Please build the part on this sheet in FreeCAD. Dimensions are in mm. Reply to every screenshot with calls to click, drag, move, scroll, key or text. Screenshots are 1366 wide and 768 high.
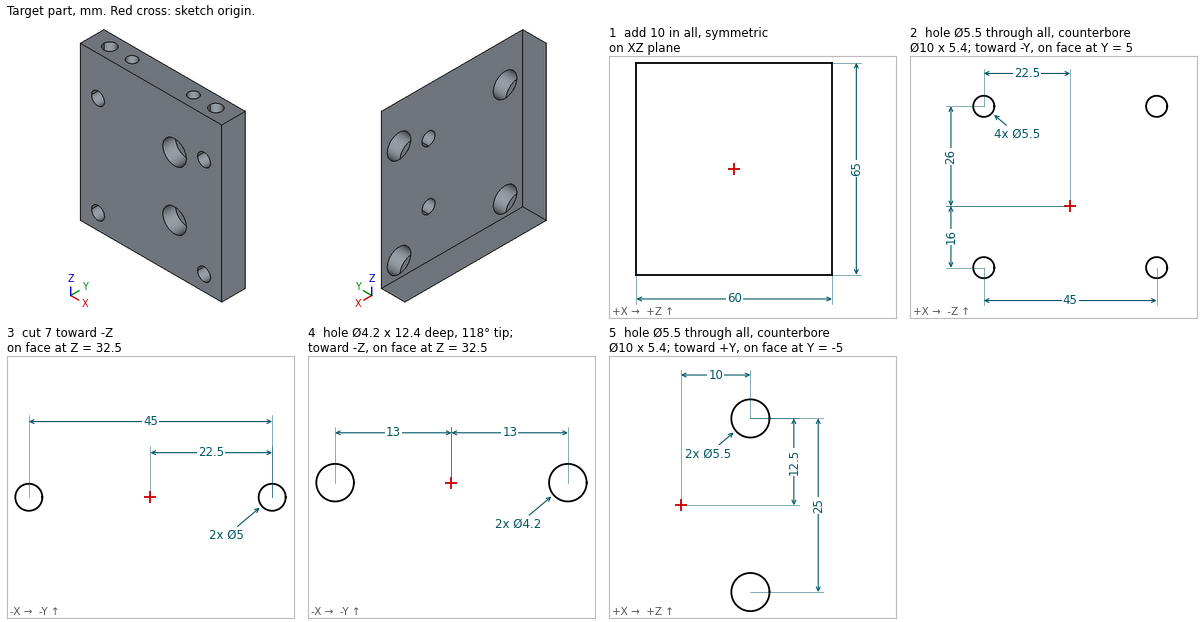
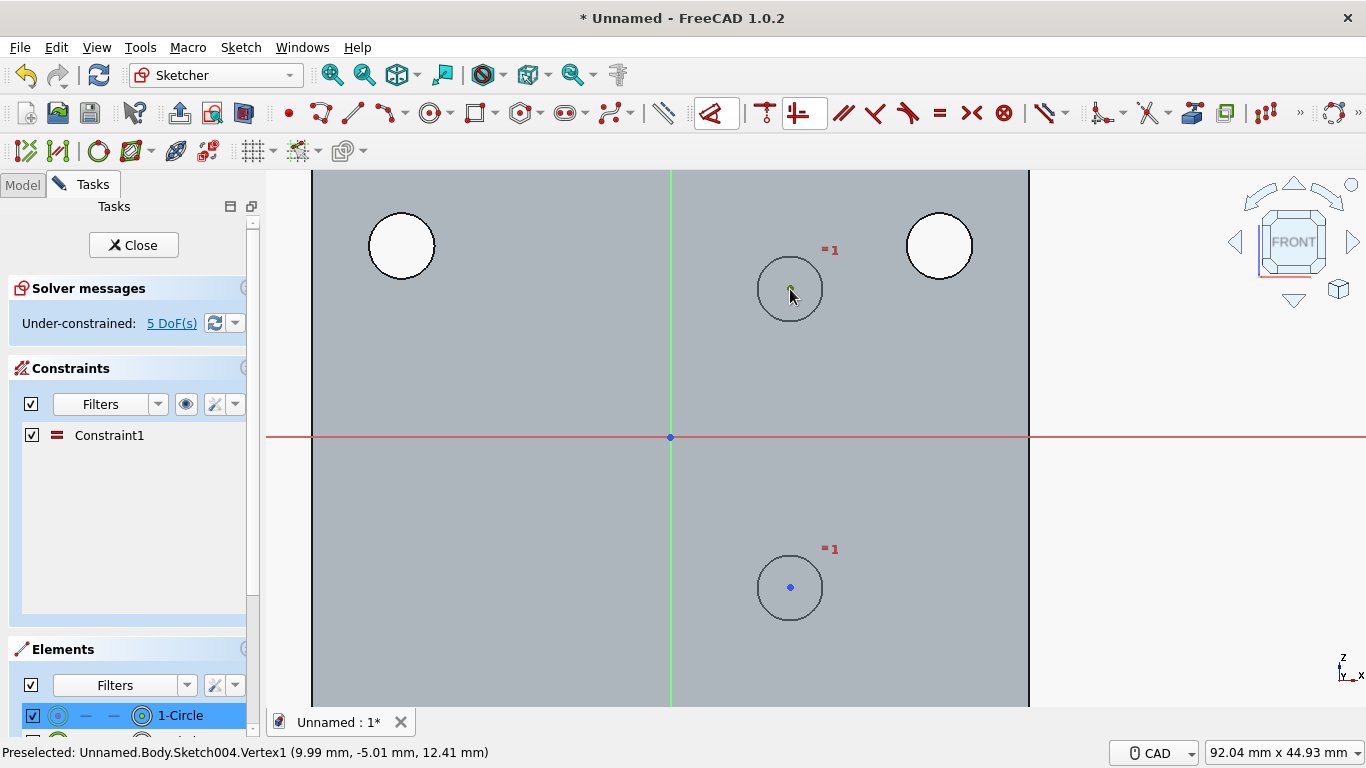
click(790, 588)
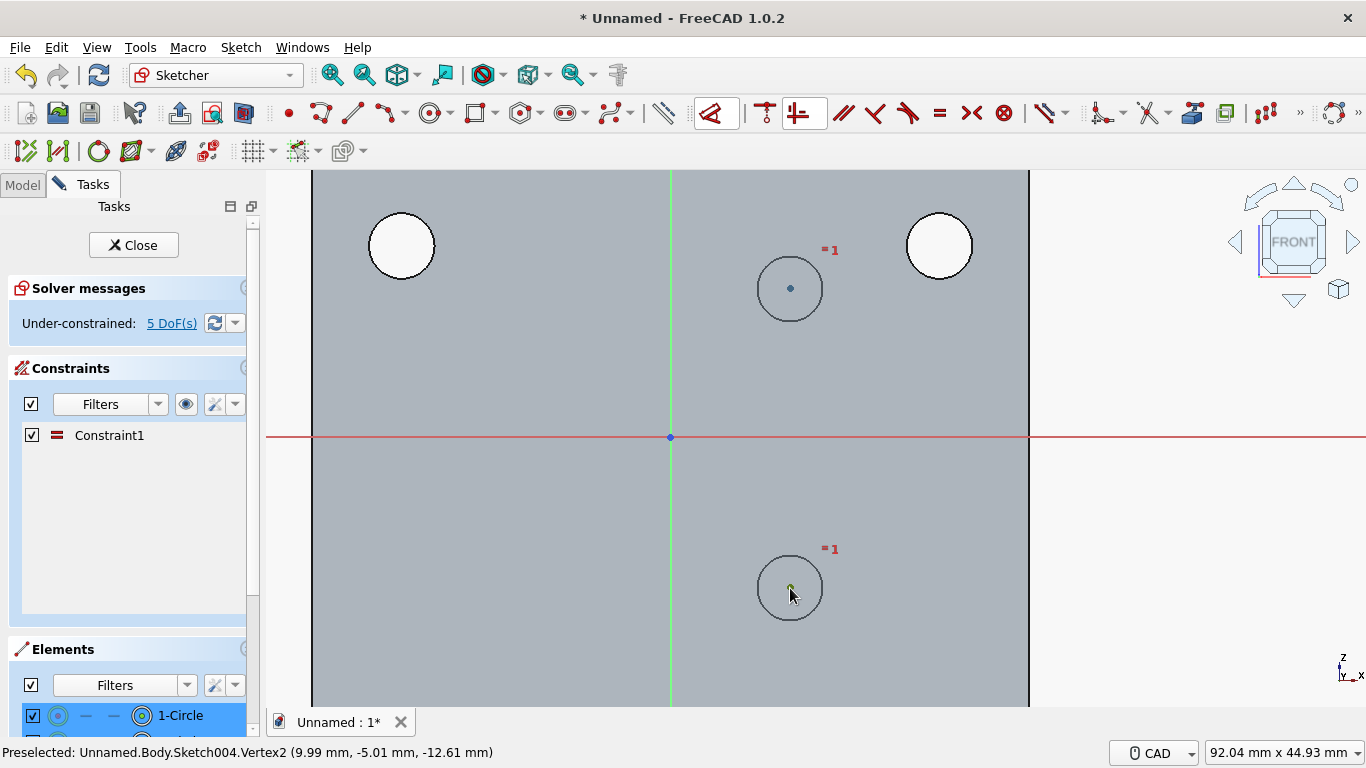
key(v)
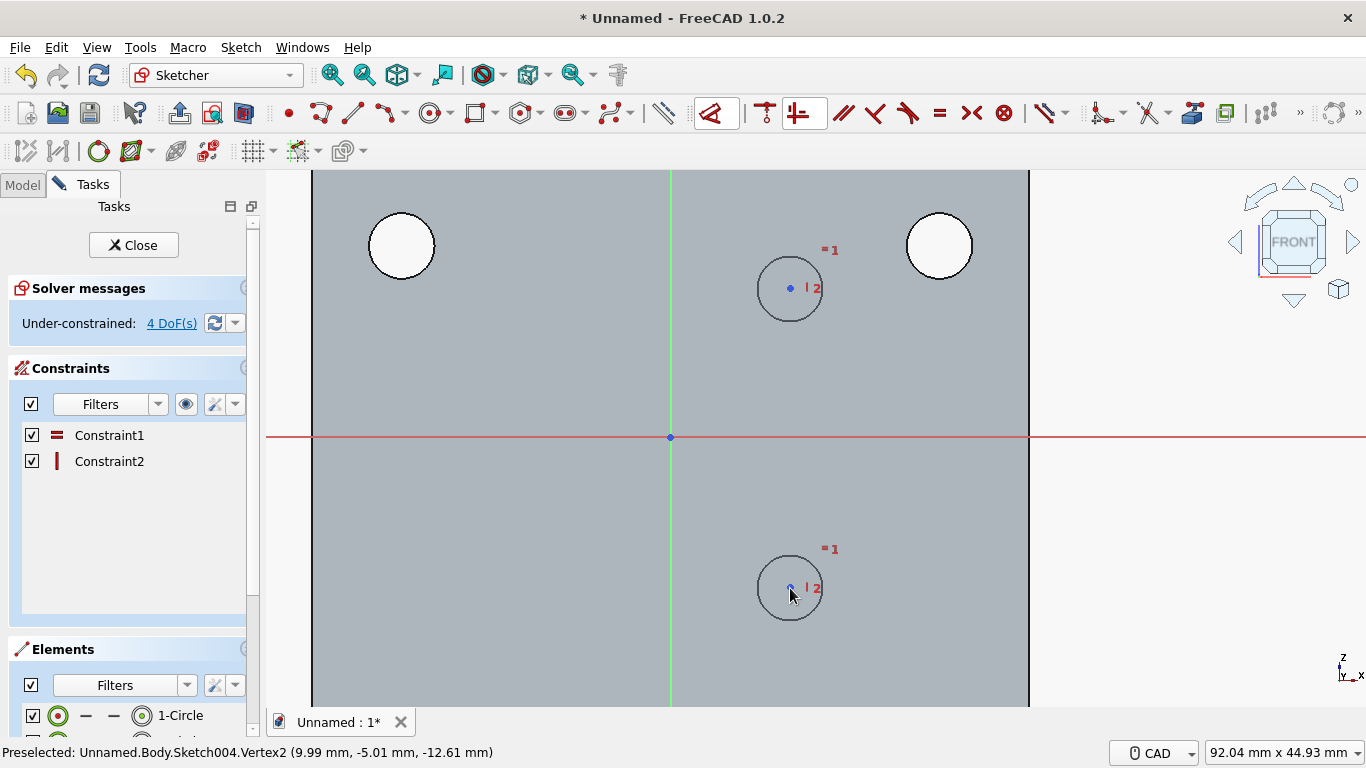
click(813, 266)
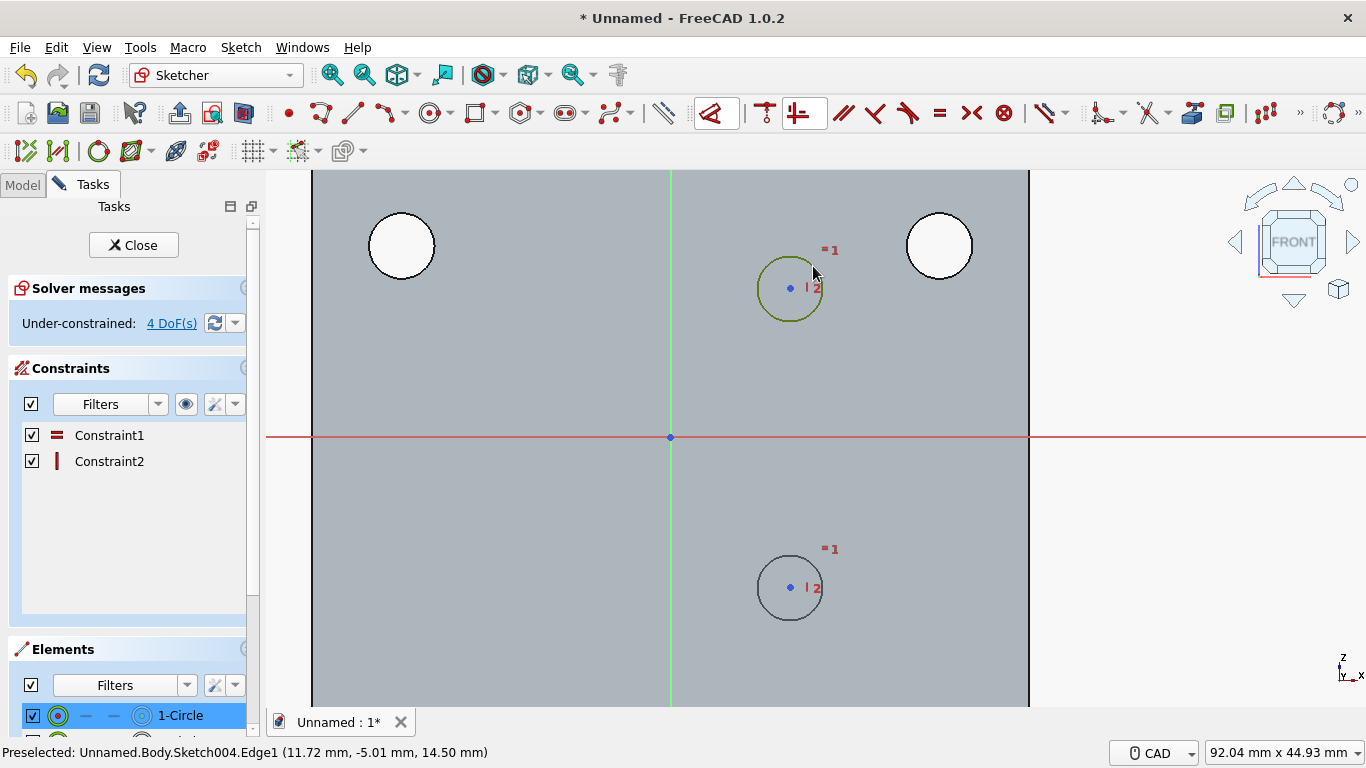
key(k)
key(o)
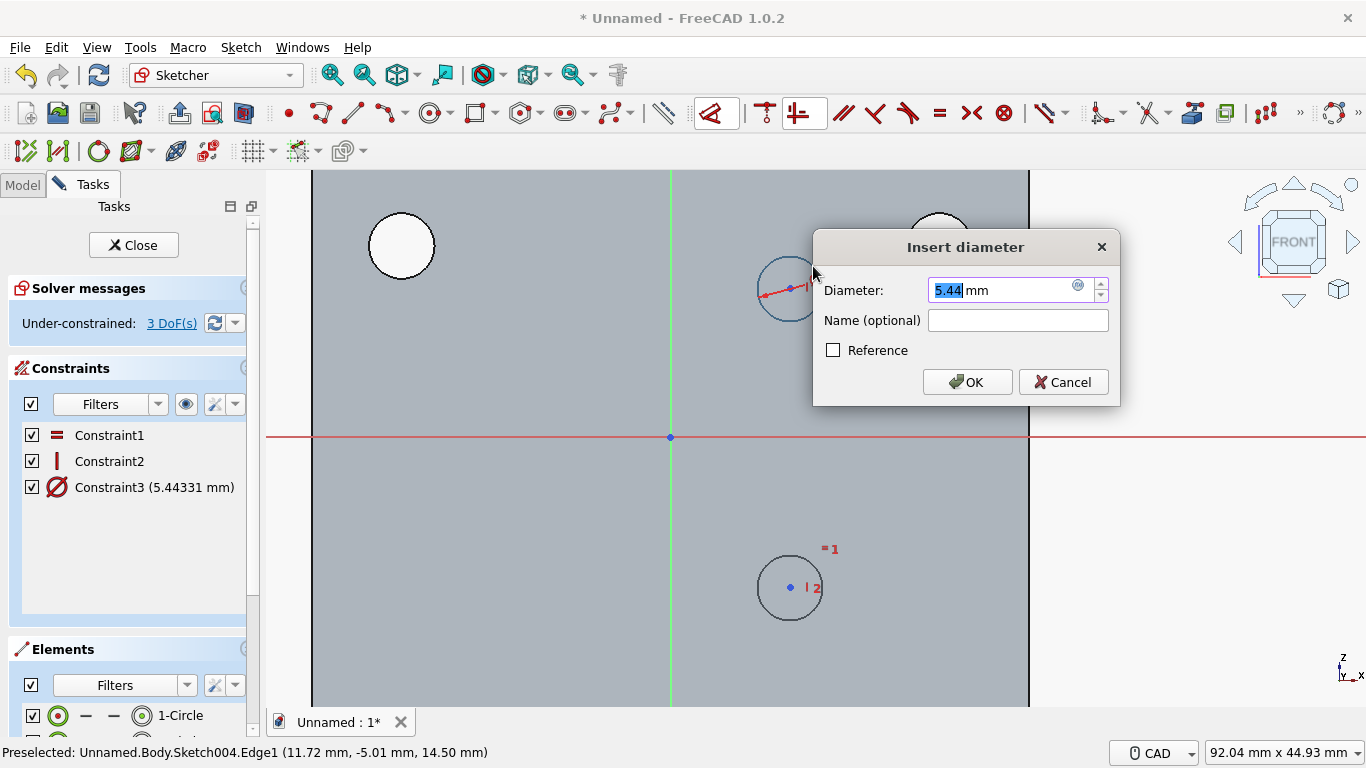
text(5.5)
key(Return)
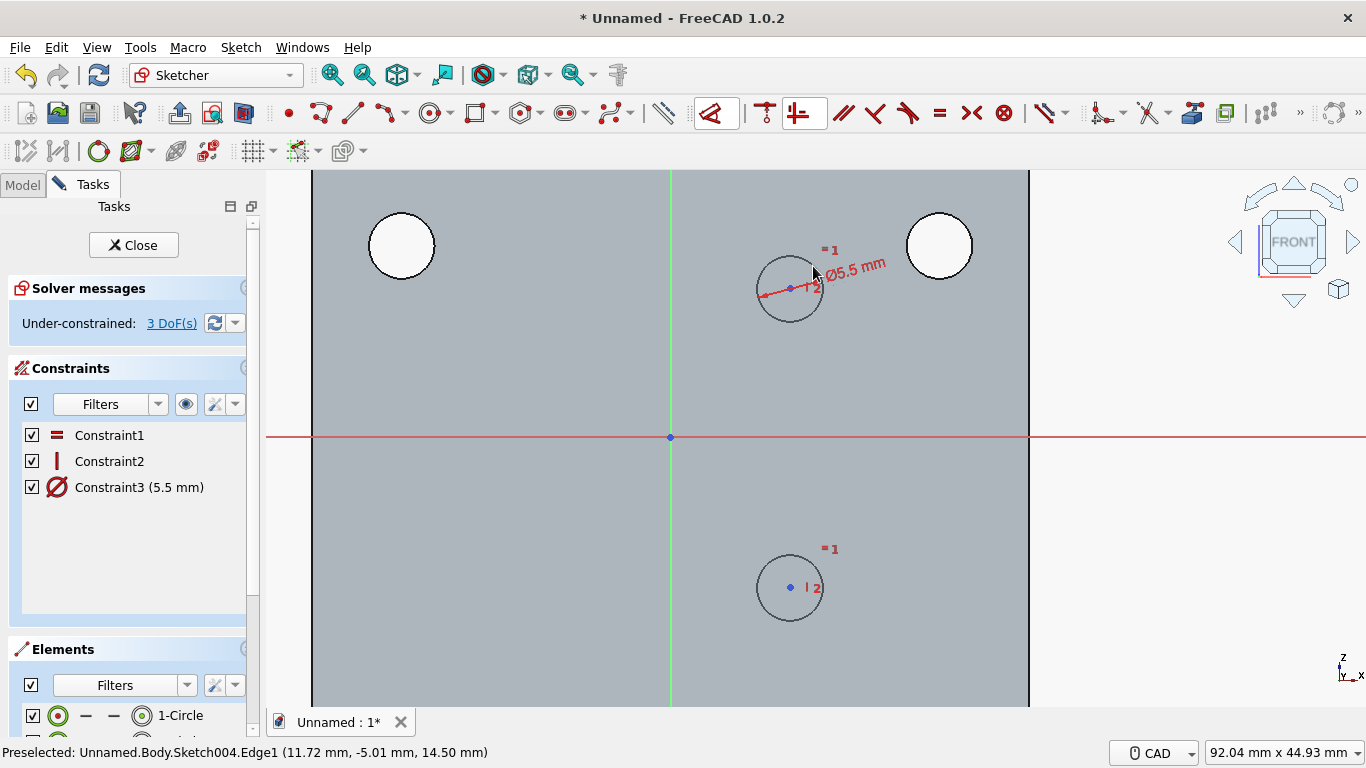
click(790, 289)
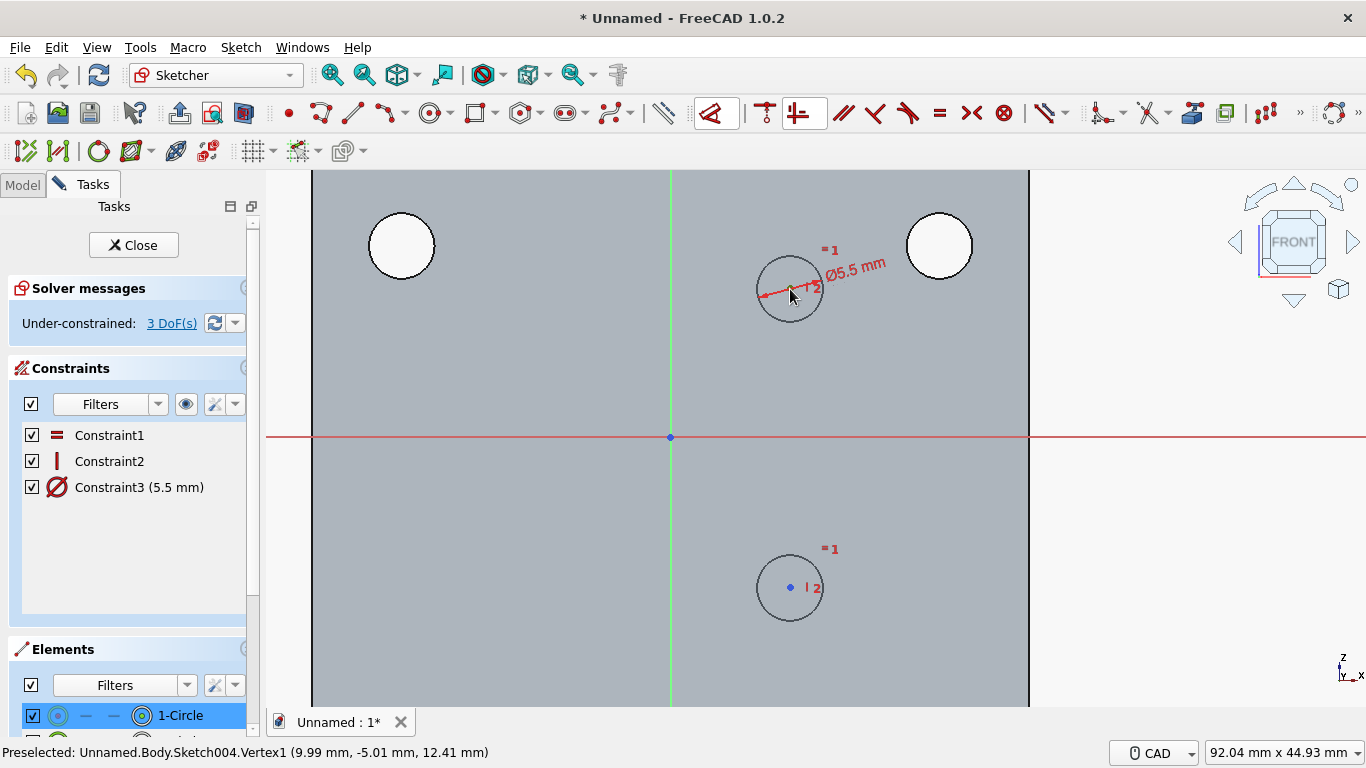
key(l)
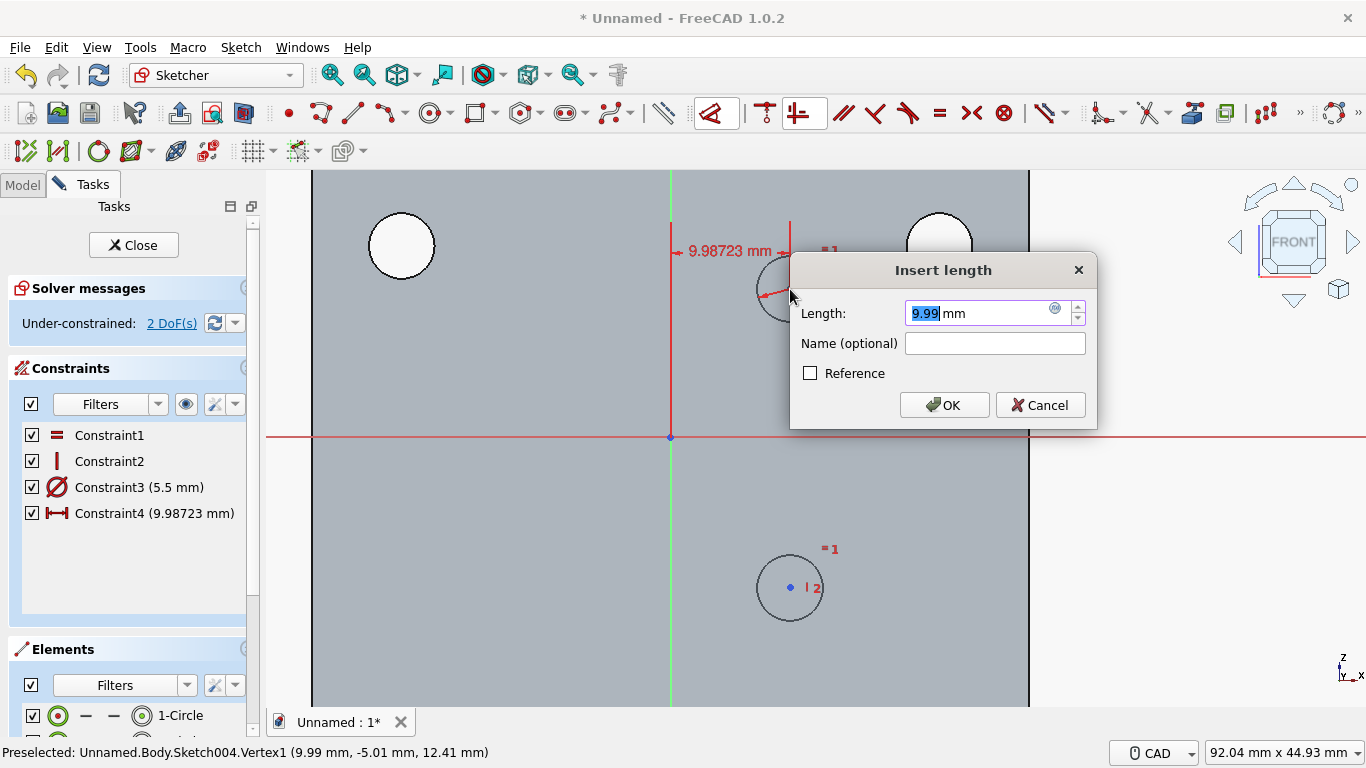
text(10)
key(Return)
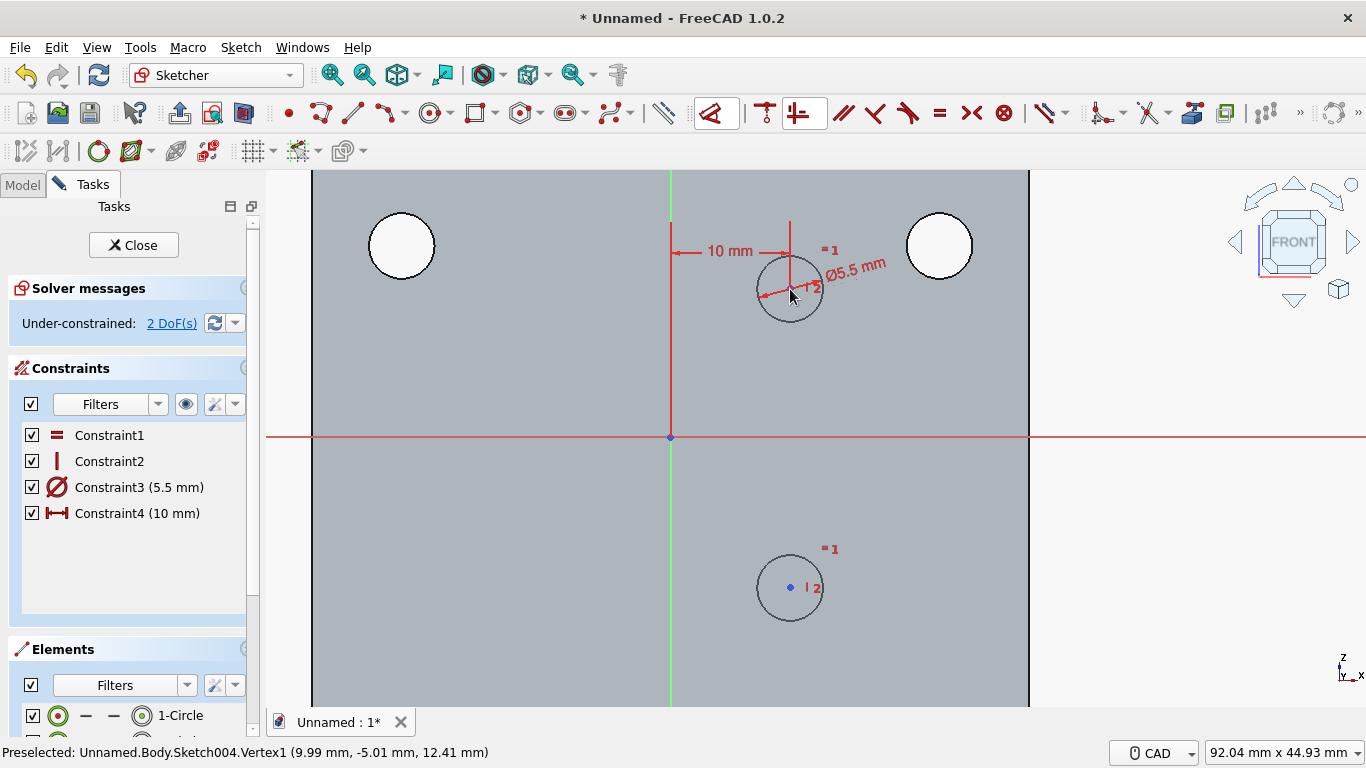
click(790, 289)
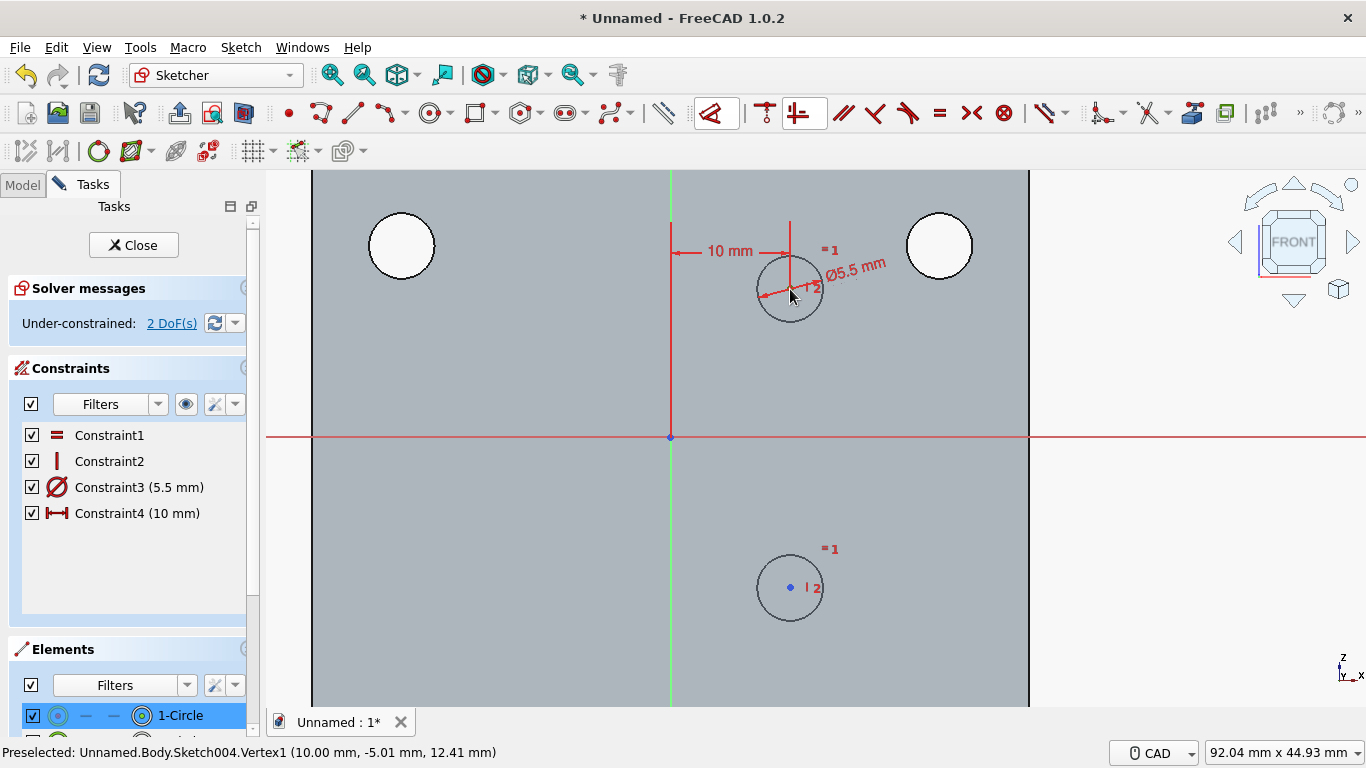
click(790, 588)